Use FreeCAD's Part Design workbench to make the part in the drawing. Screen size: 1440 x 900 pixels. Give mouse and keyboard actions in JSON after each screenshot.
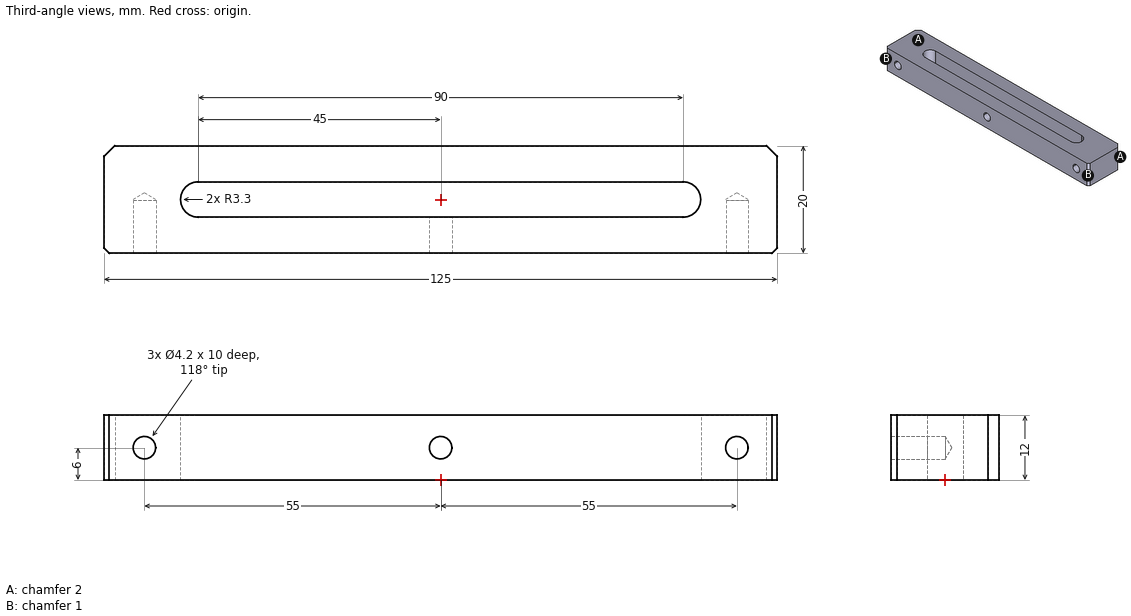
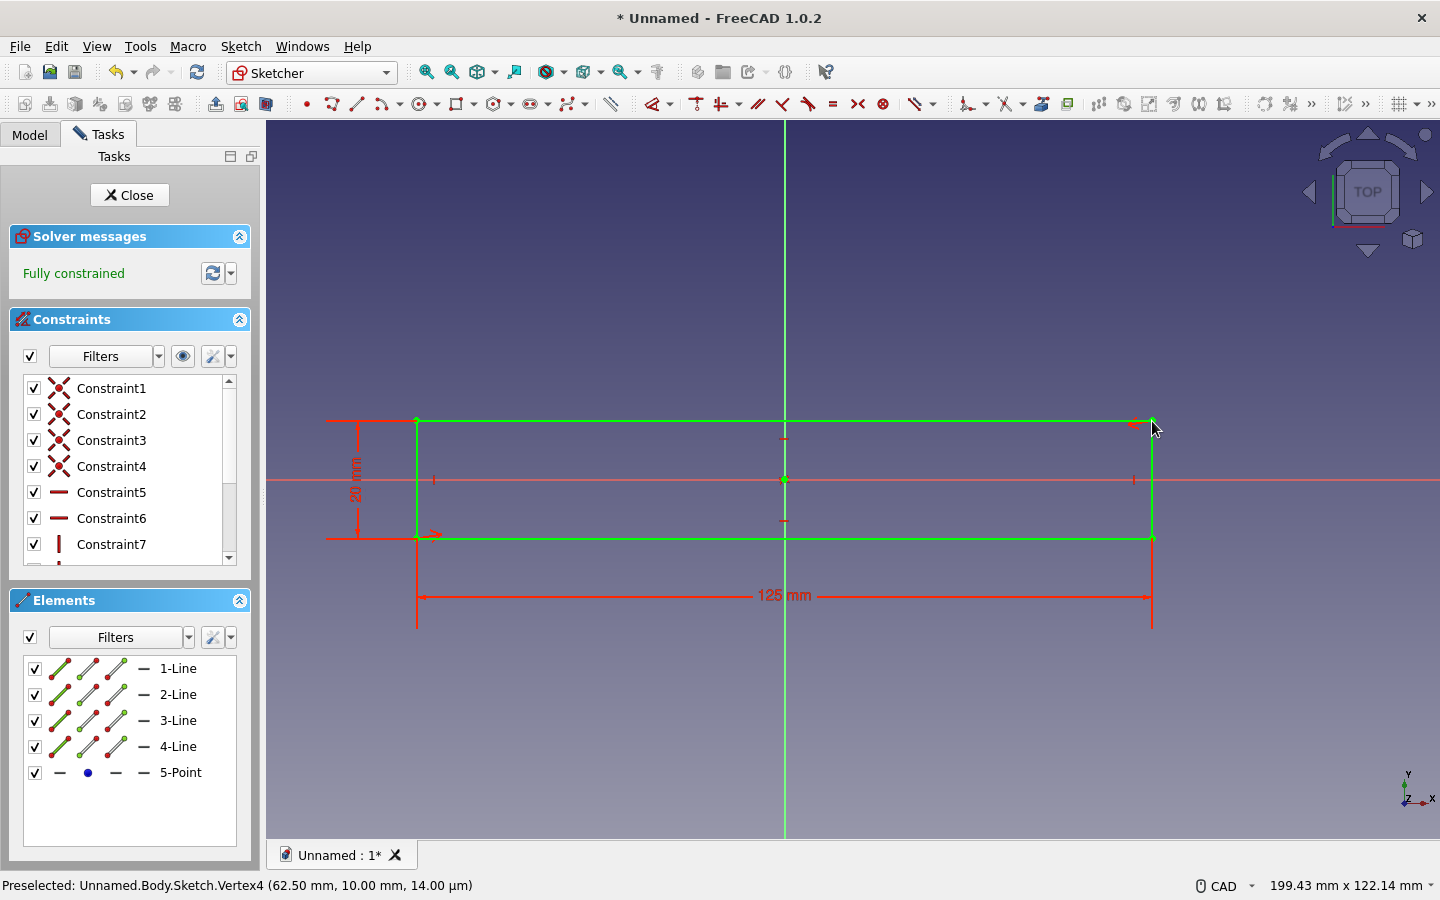
{"action": "left_click", "coordinate": [130, 195]}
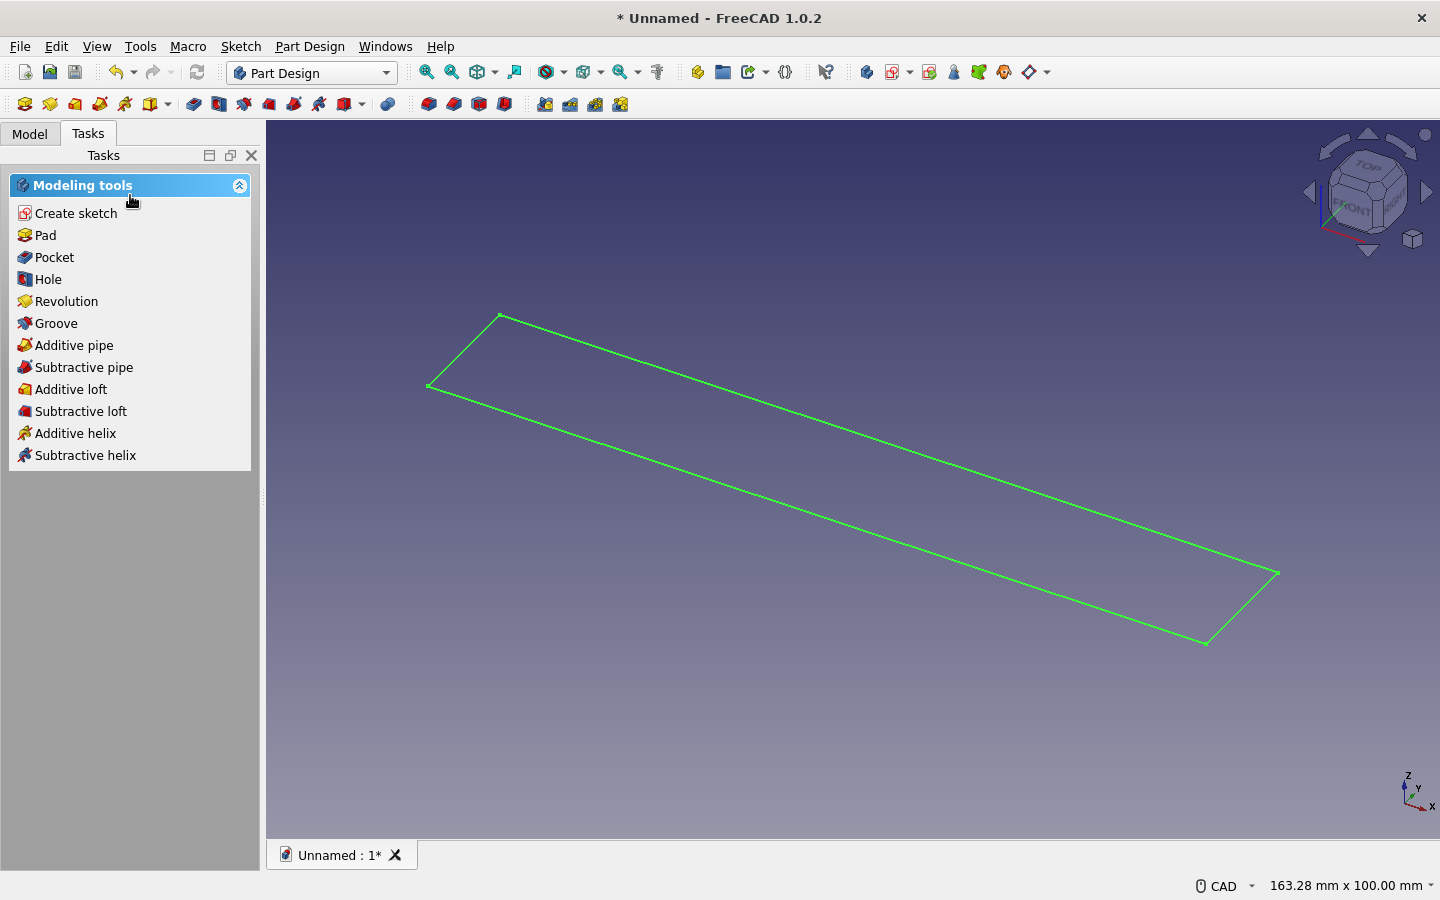
{"action": "left_click", "coordinate": [25, 104]}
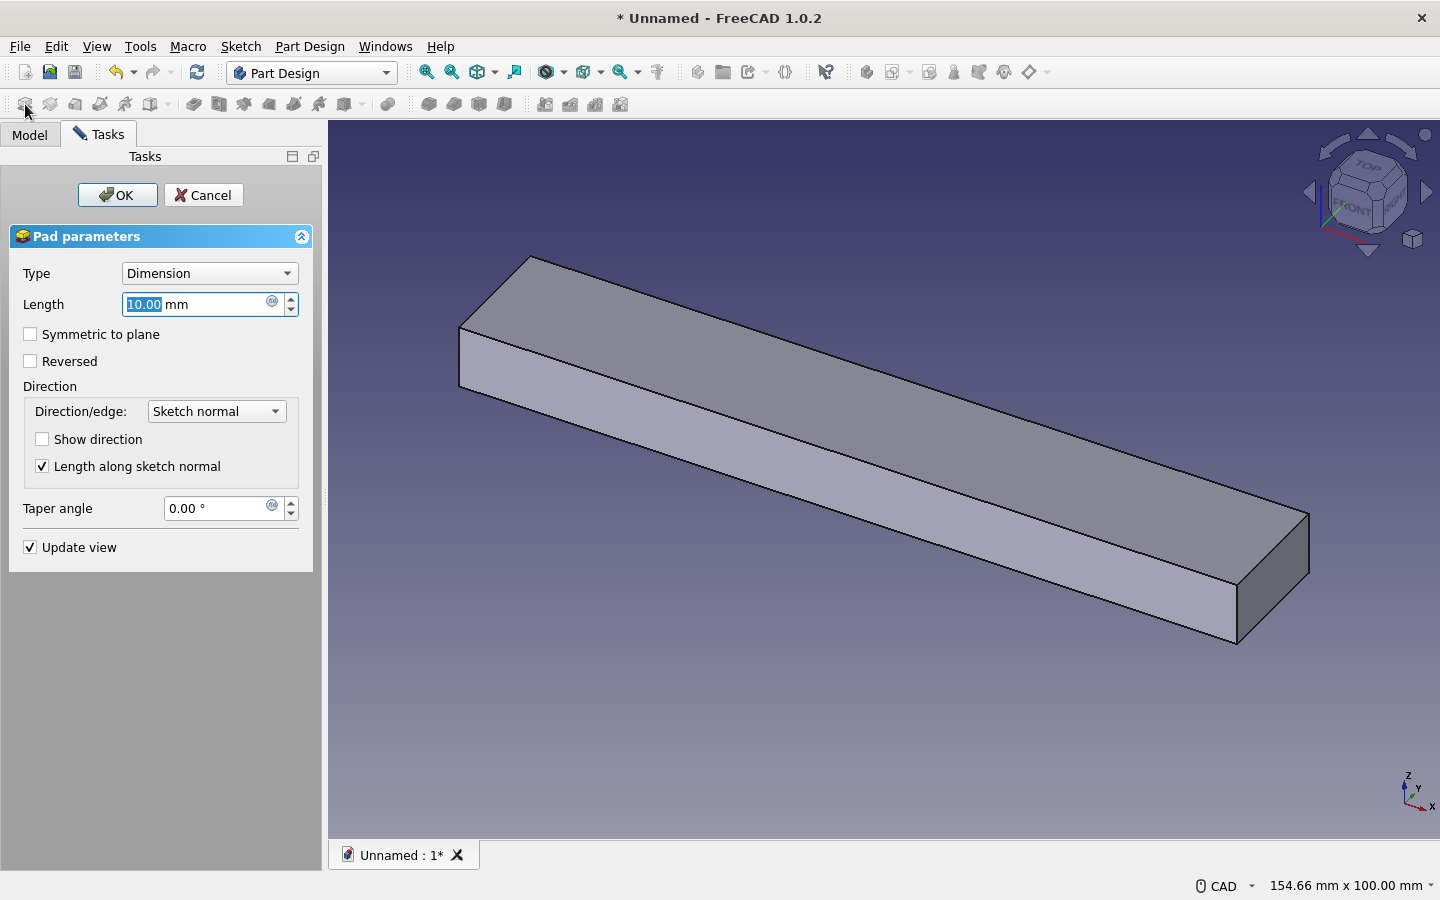
{"action": "type", "text": "12"}
{"action": "key", "text": "Tab"}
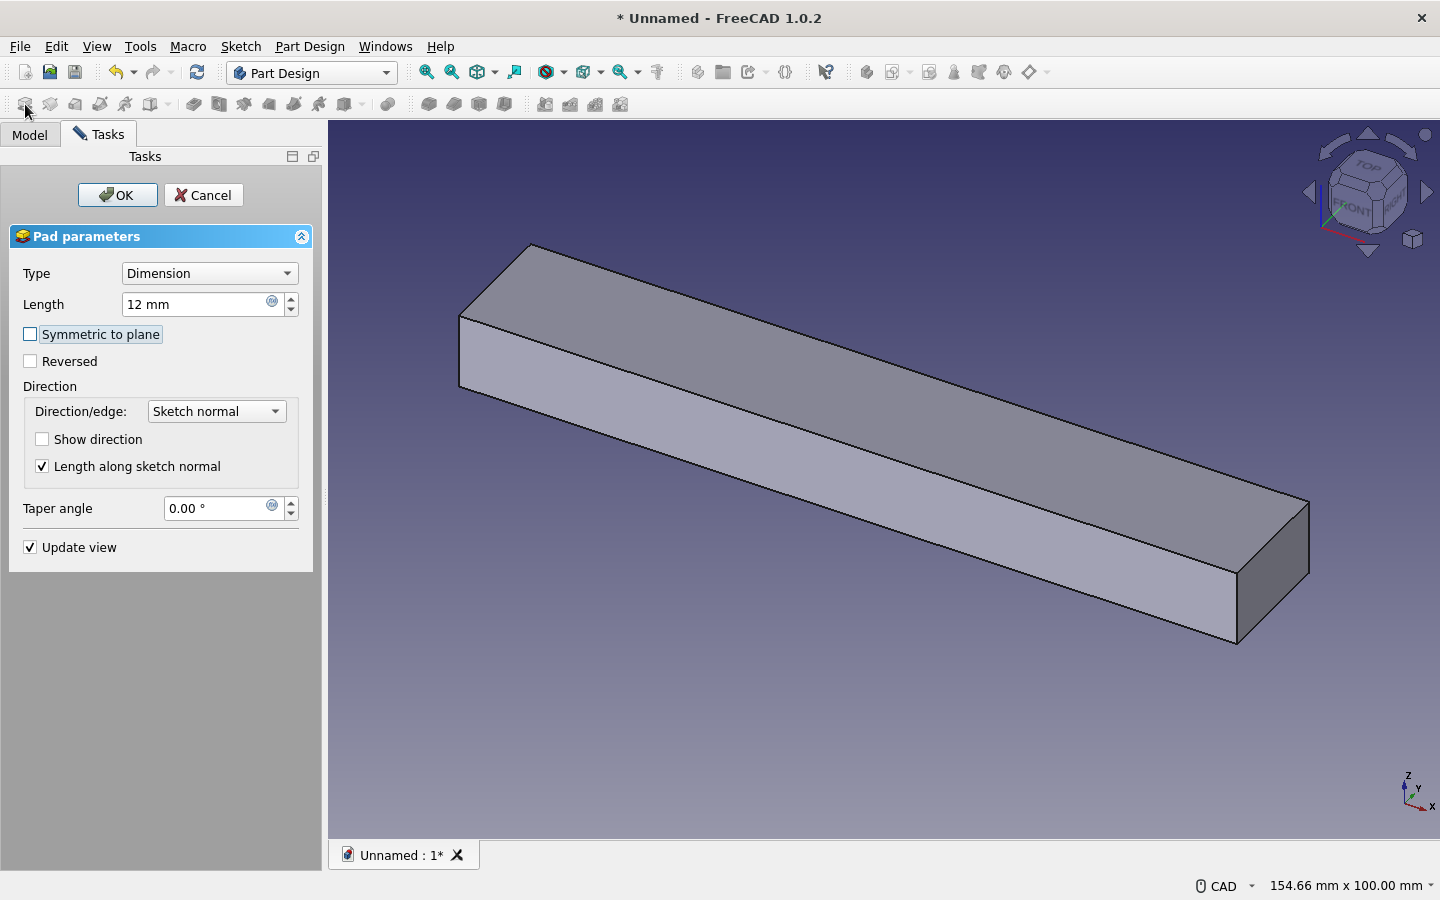
{"action": "left_click", "coordinate": [118, 195]}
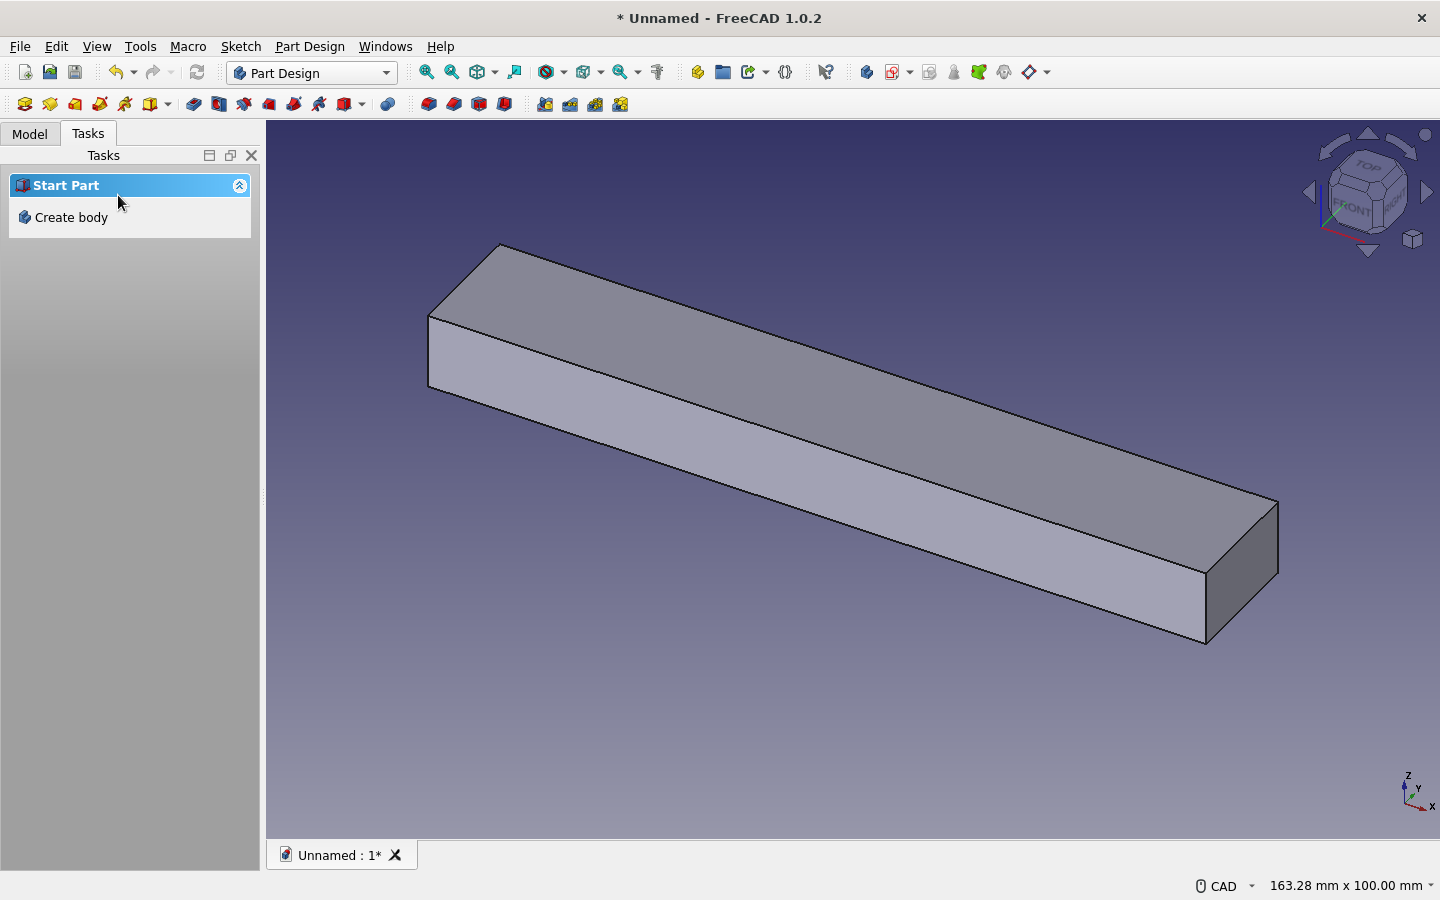
{"action": "left_click", "coordinate": [1075, 481]}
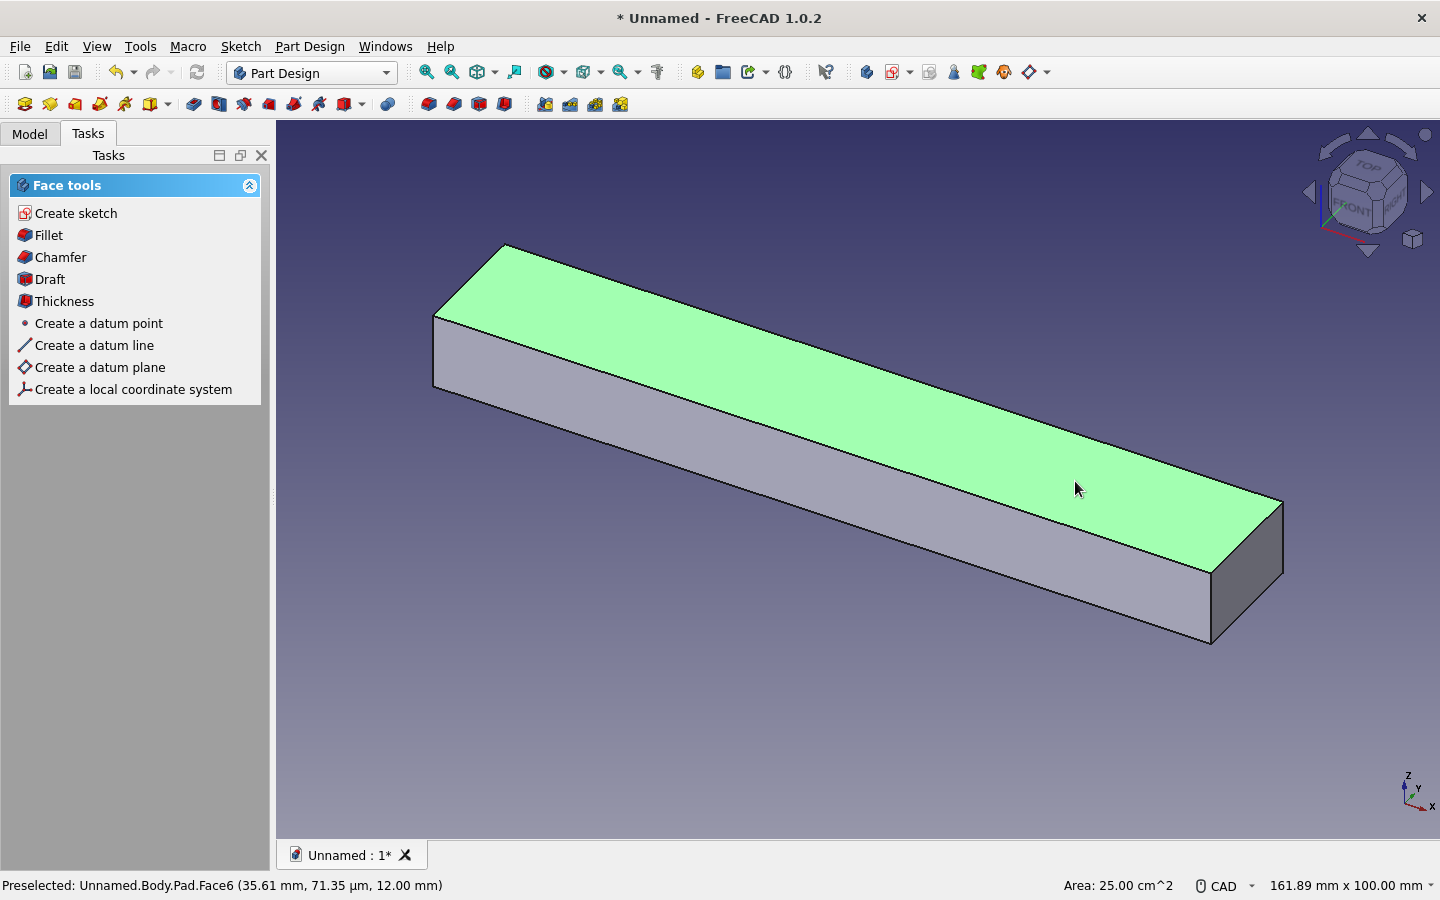
{"action": "left_click", "coordinate": [892, 72]}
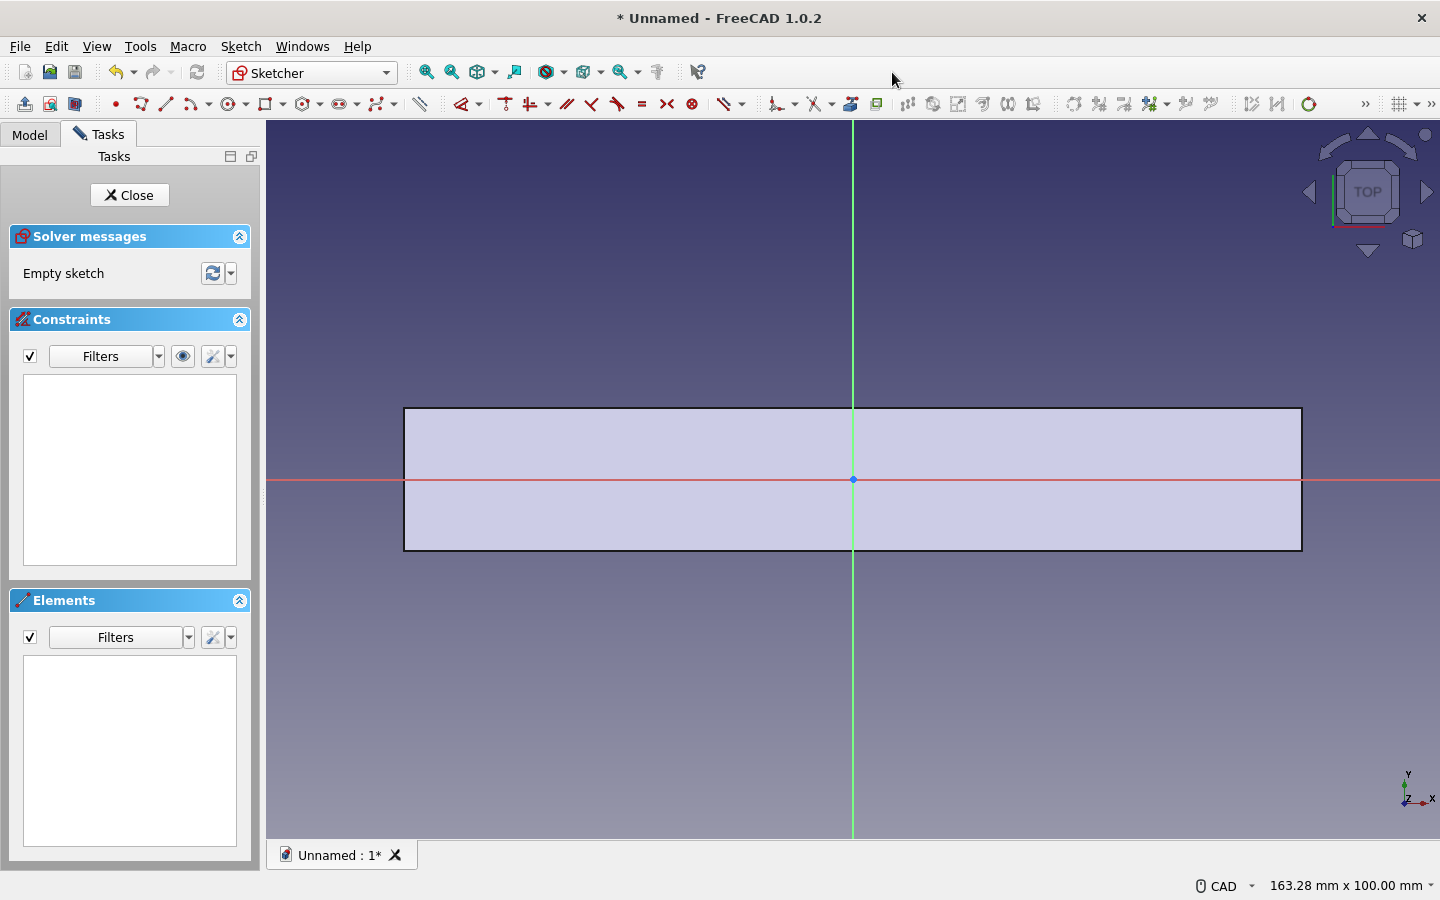
{"action": "key", "text": "g s"}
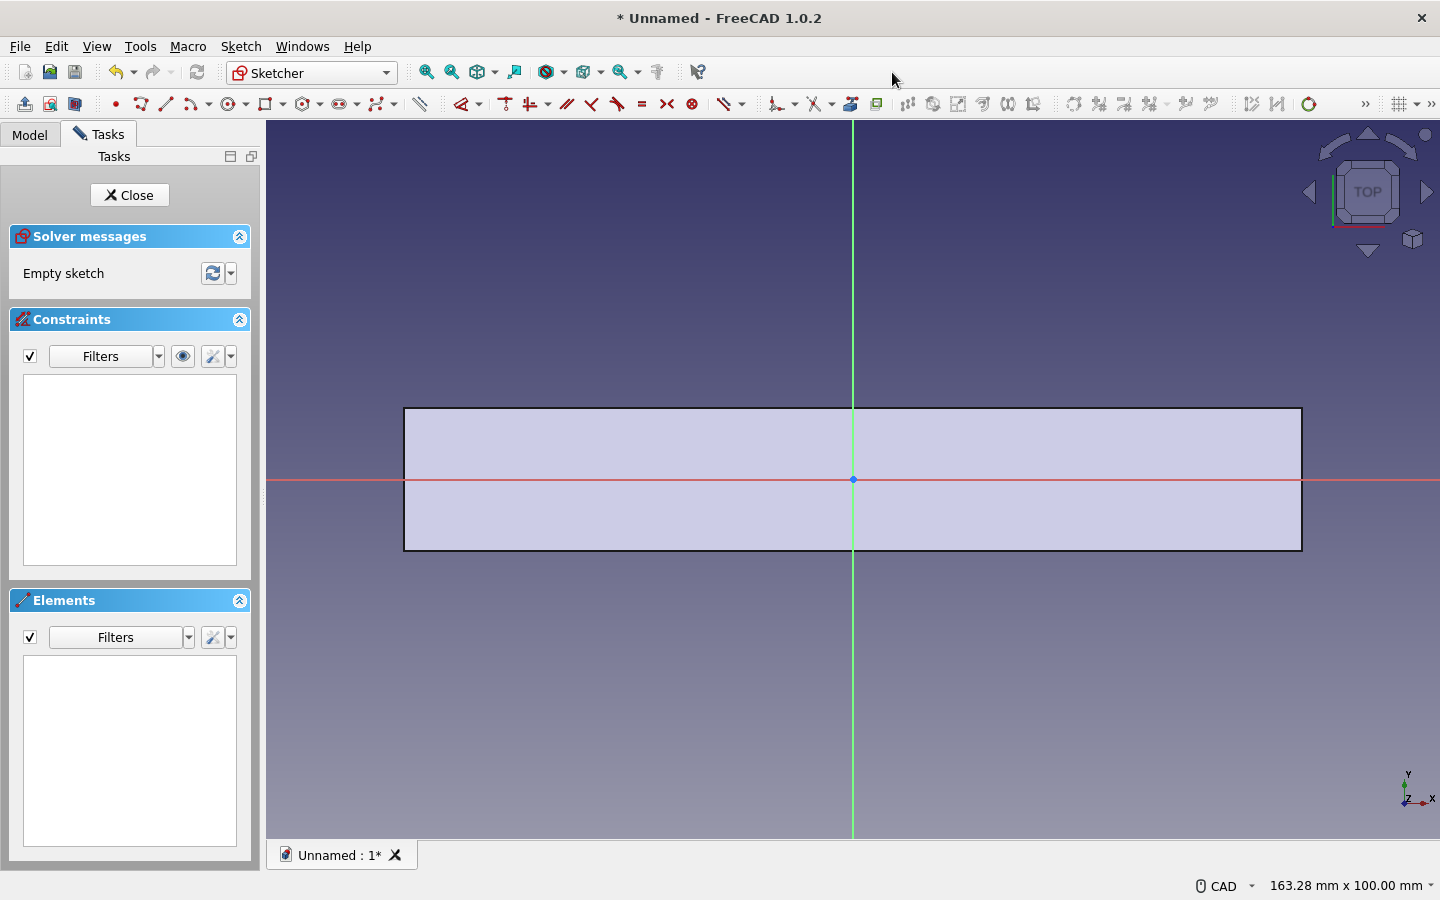
{"action": "left_click", "coordinate": [529, 480]}